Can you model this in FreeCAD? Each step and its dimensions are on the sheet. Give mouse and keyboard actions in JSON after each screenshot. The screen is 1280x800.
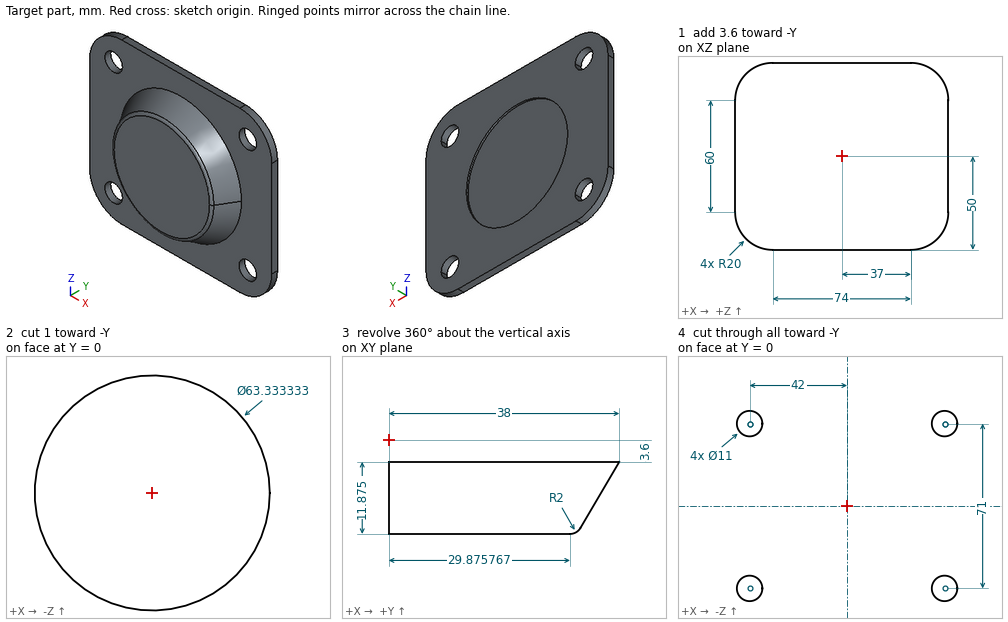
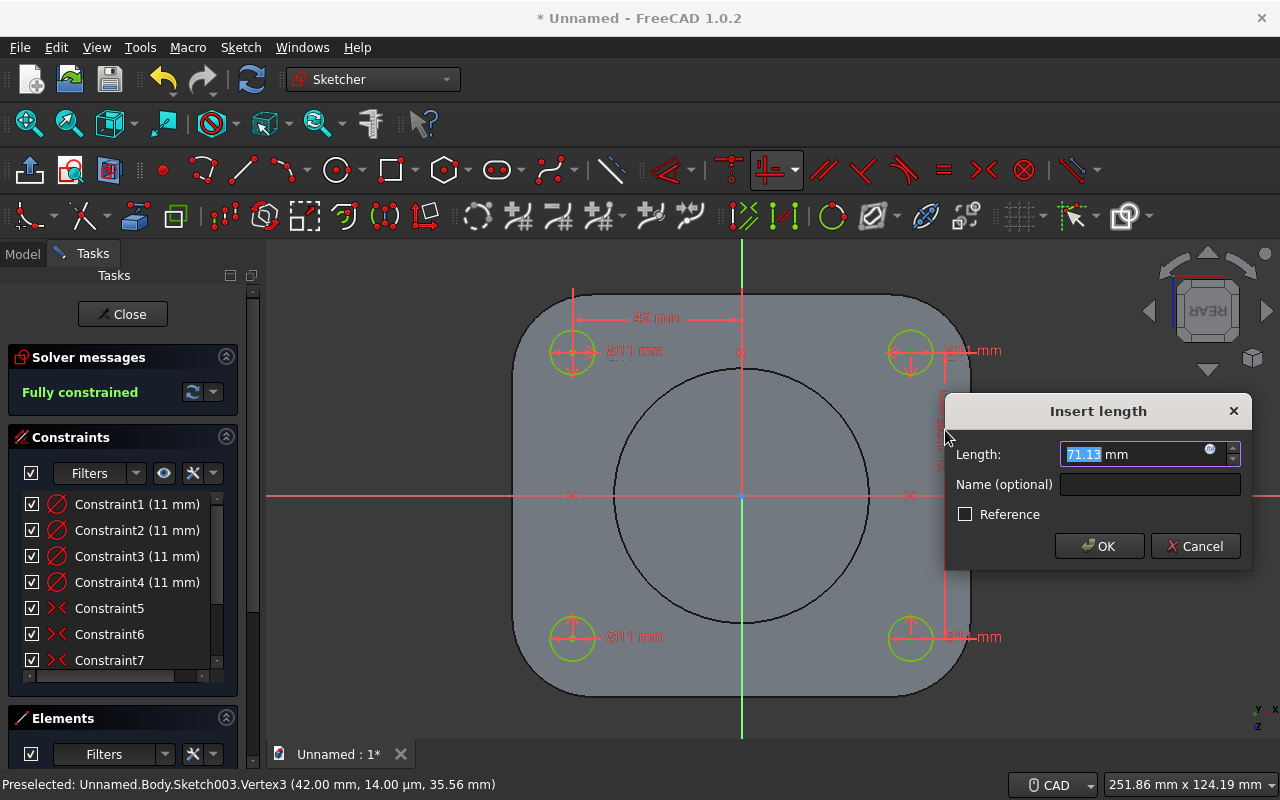
{"action": "type", "text": "71"}
{"action": "key", "text": "Return"}
{"action": "key", "text": "Escape"}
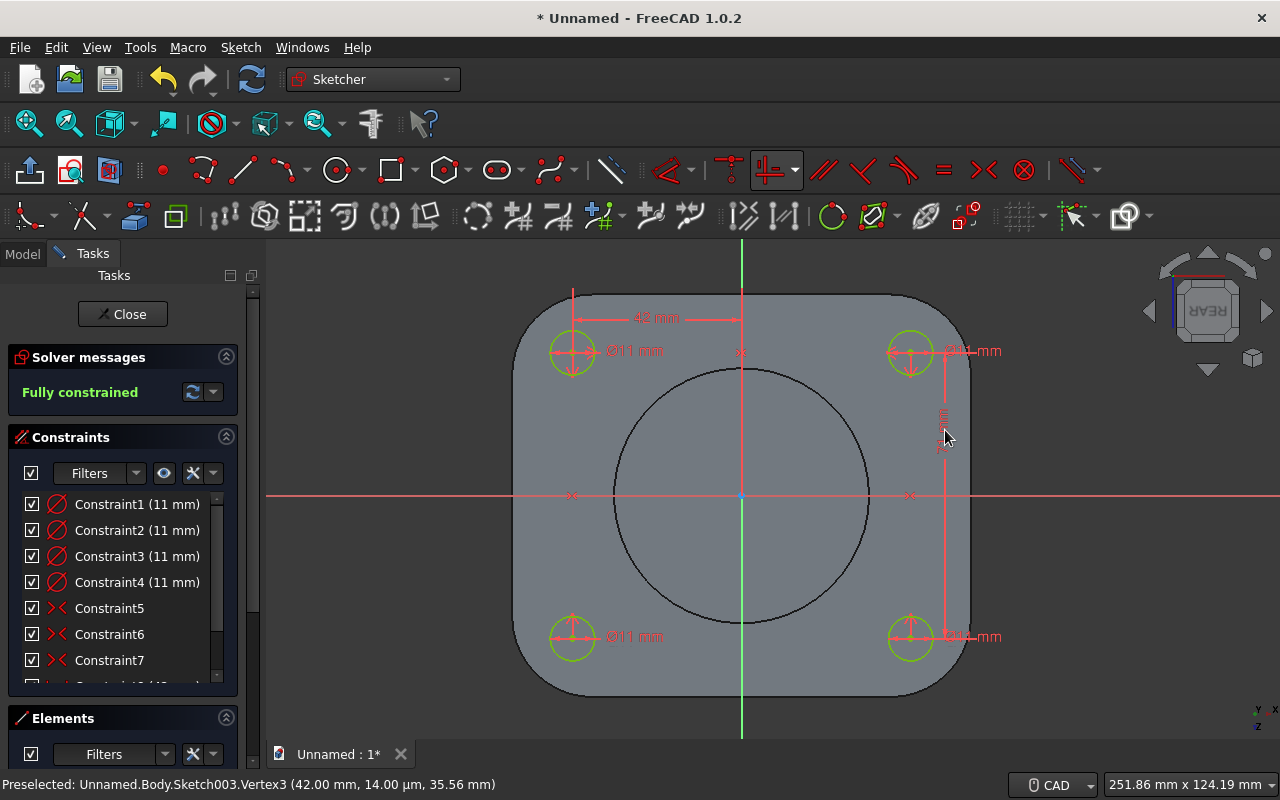
{"action": "left_click", "coordinate": [123, 314]}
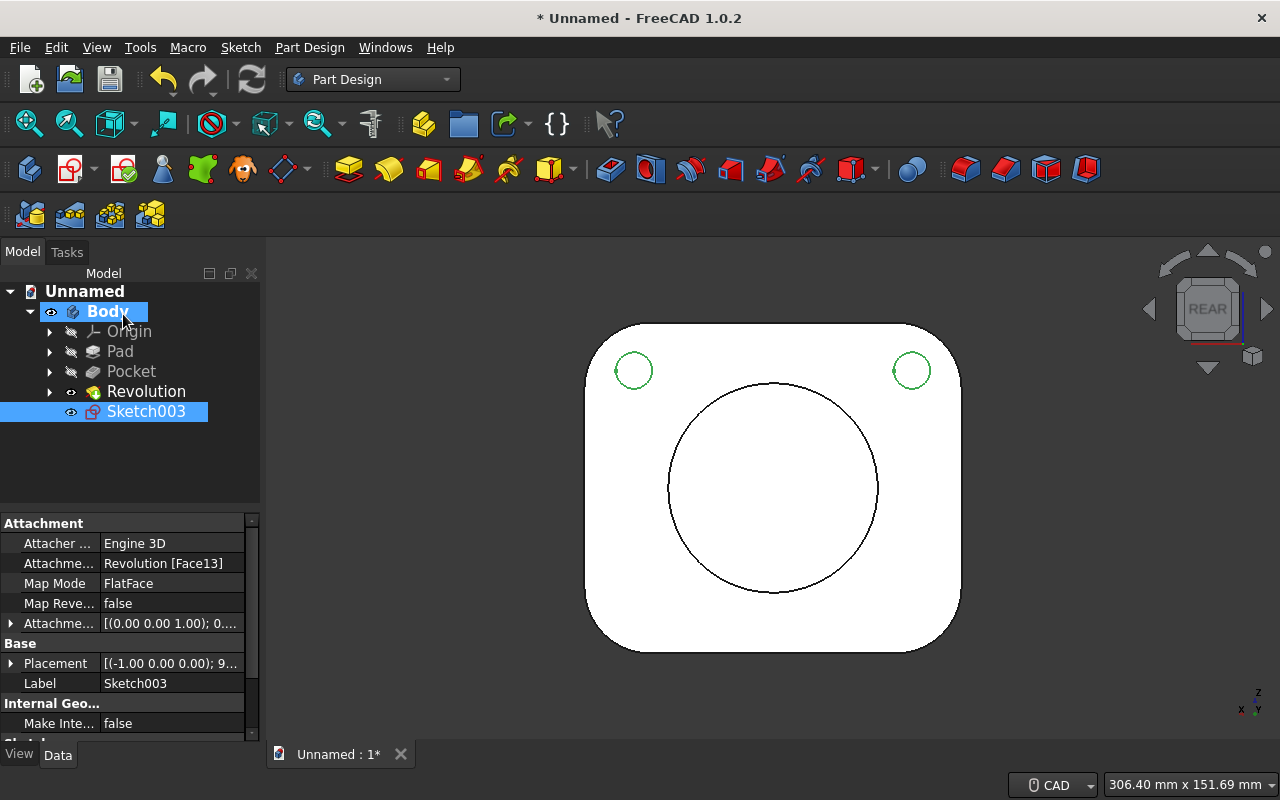
{"action": "left_click", "coordinate": [612, 170]}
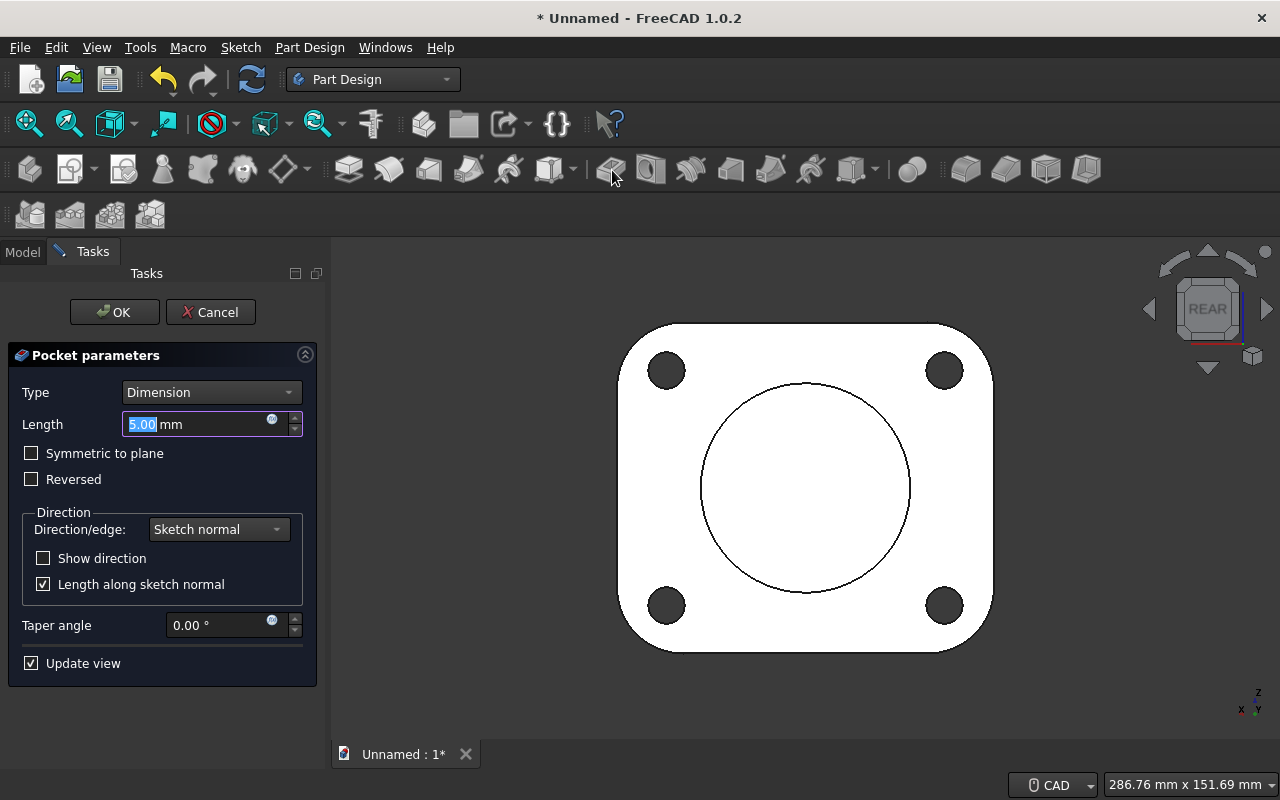
{"action": "left_click", "coordinate": [212, 392]}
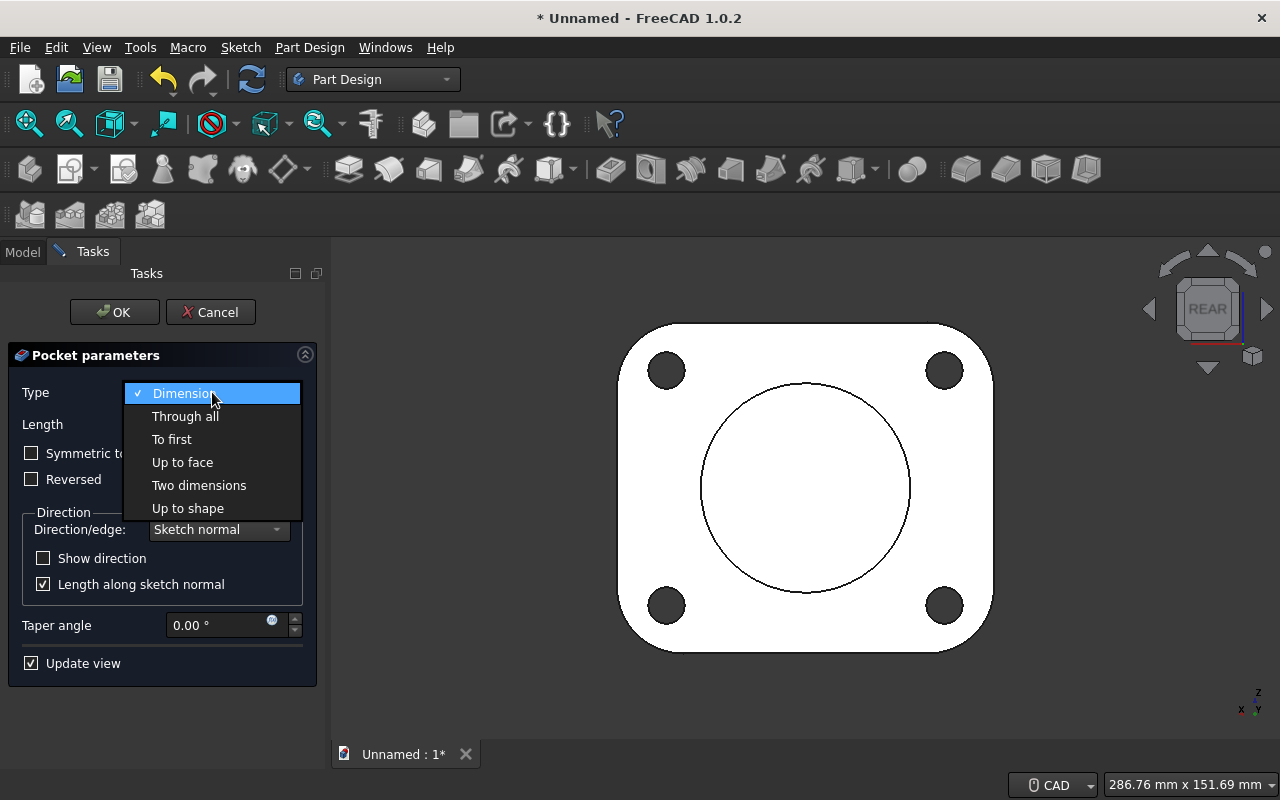
{"action": "left_click", "coordinate": [212, 416]}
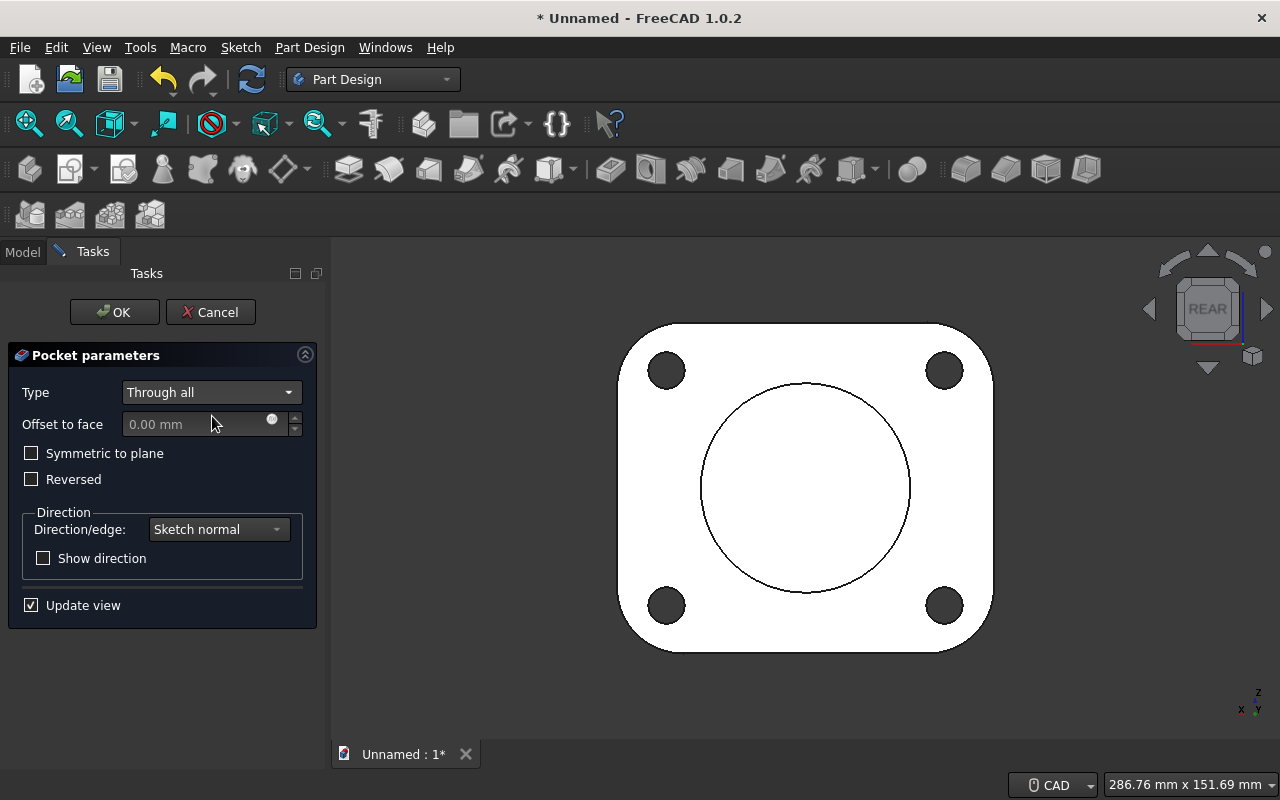
{"action": "left_click", "coordinate": [115, 312]}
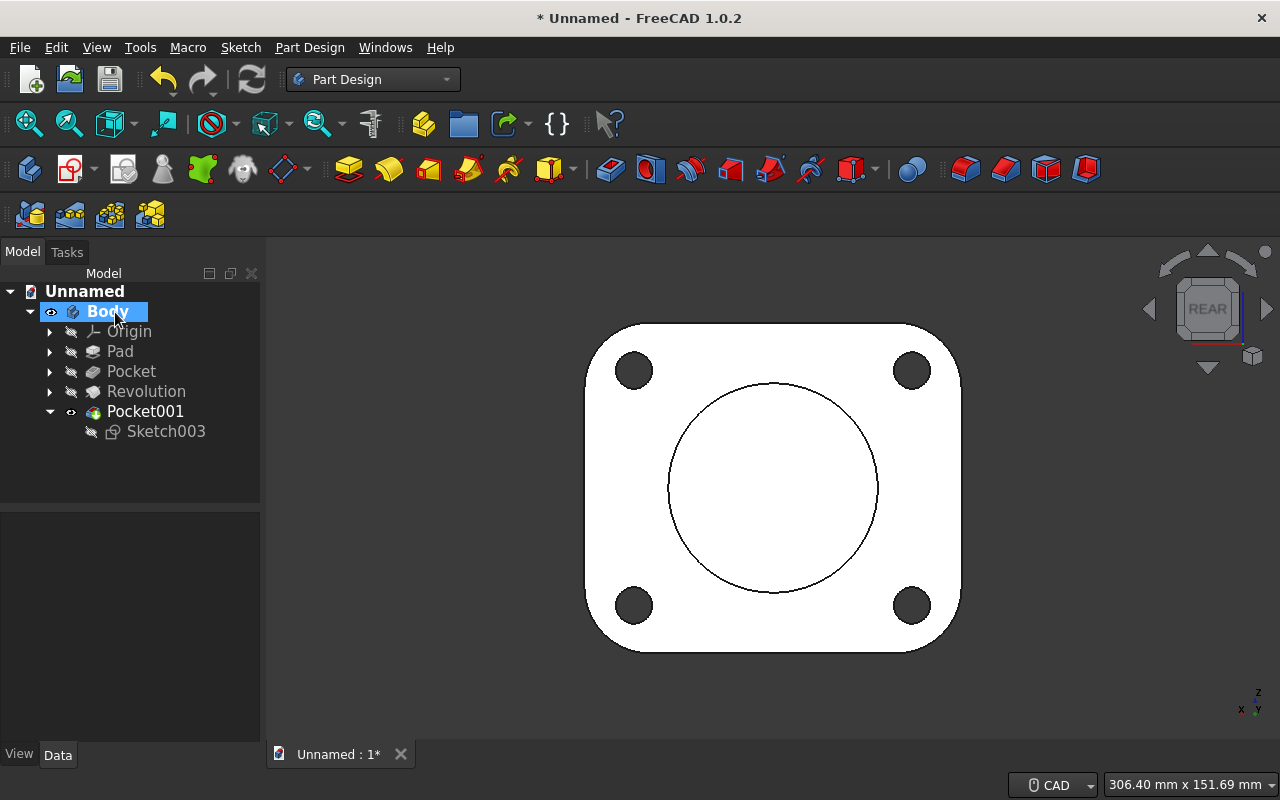
{"action": "key", "text": "0"}